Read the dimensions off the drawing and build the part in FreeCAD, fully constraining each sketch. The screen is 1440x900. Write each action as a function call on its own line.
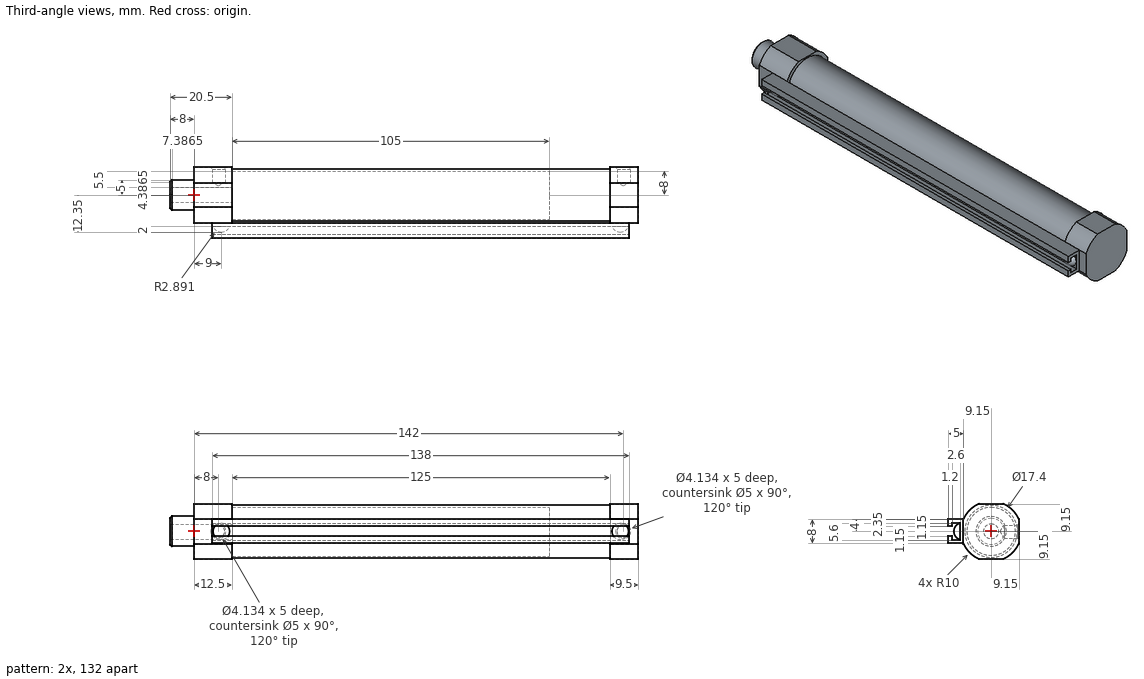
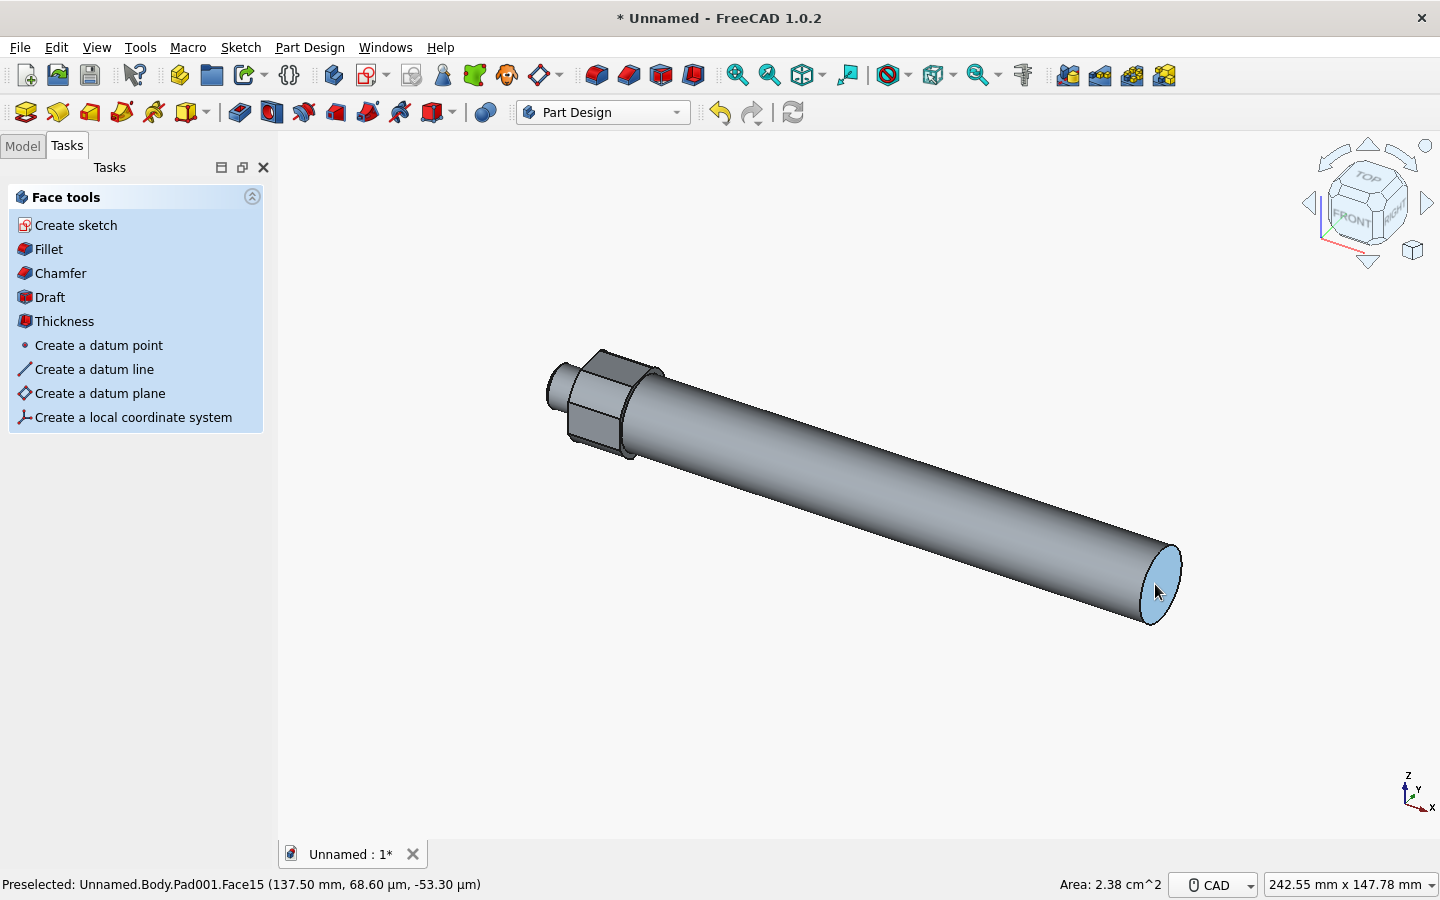
click(366, 76)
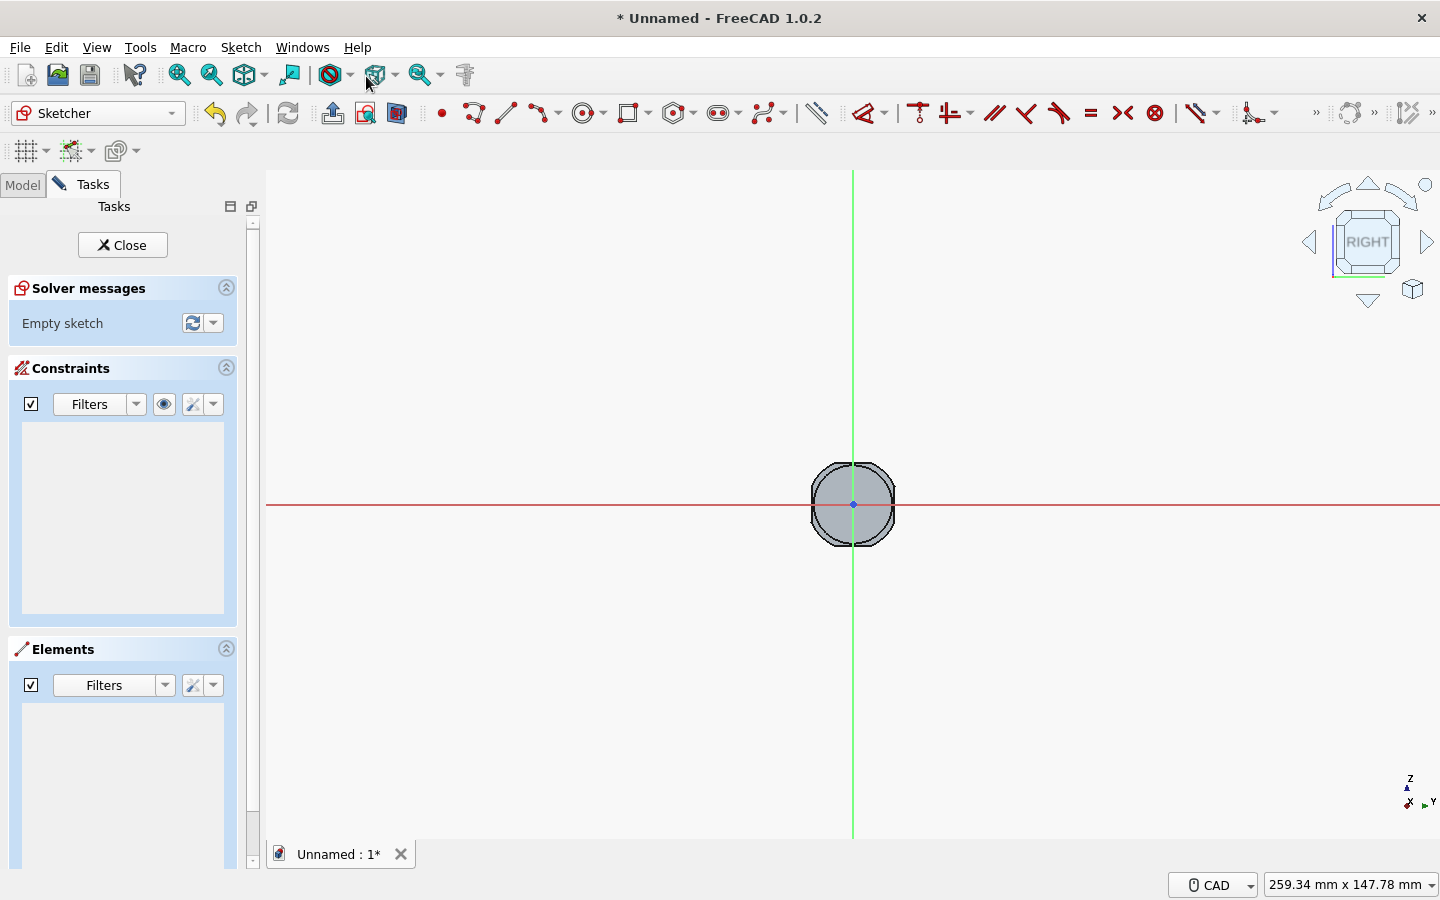
scroll(870, 504, up, 8)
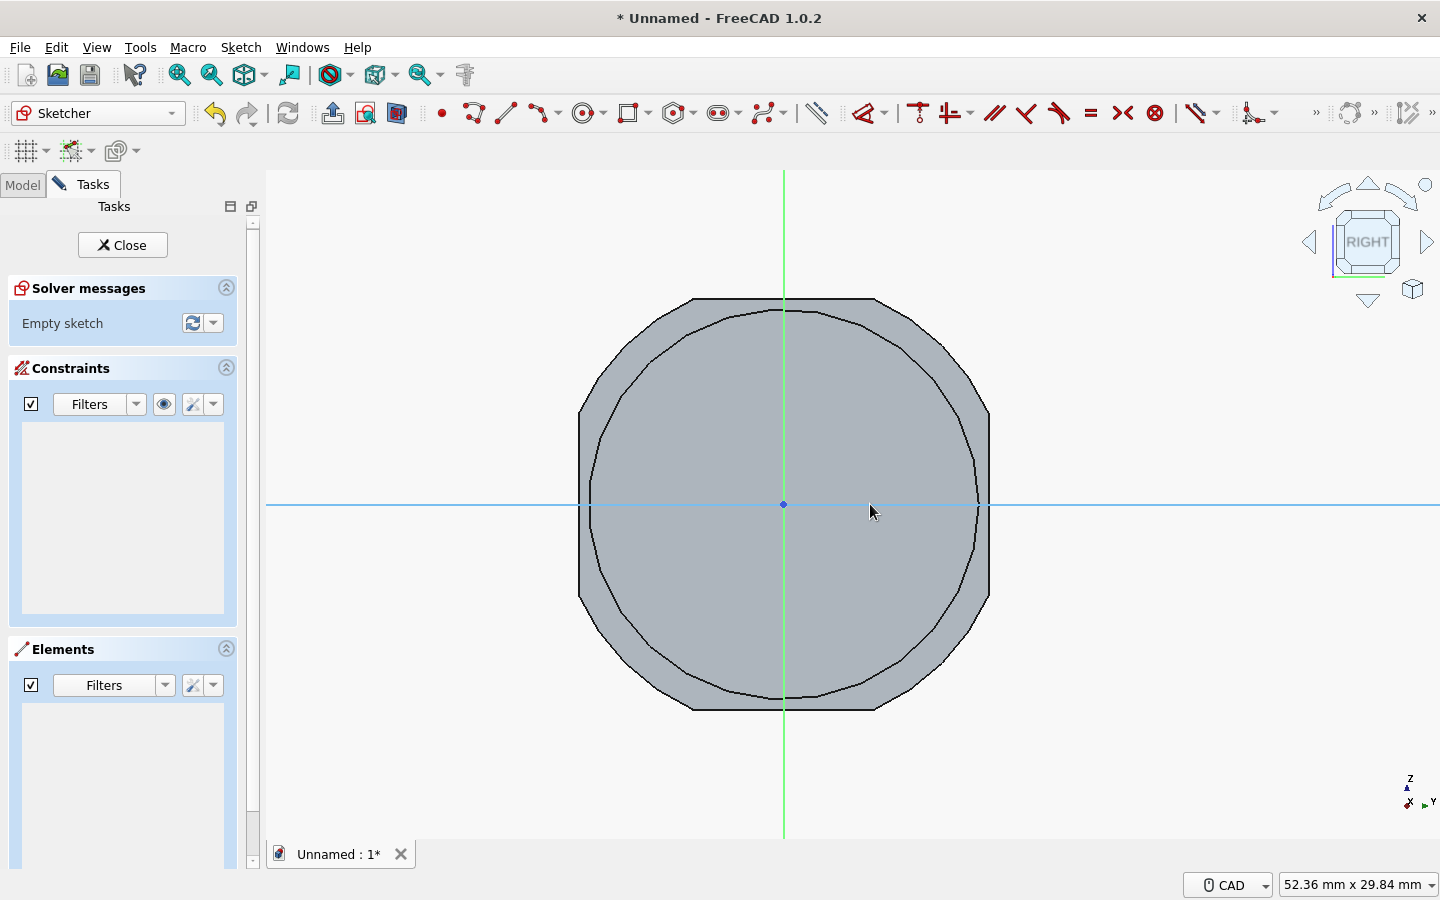
click(506, 114)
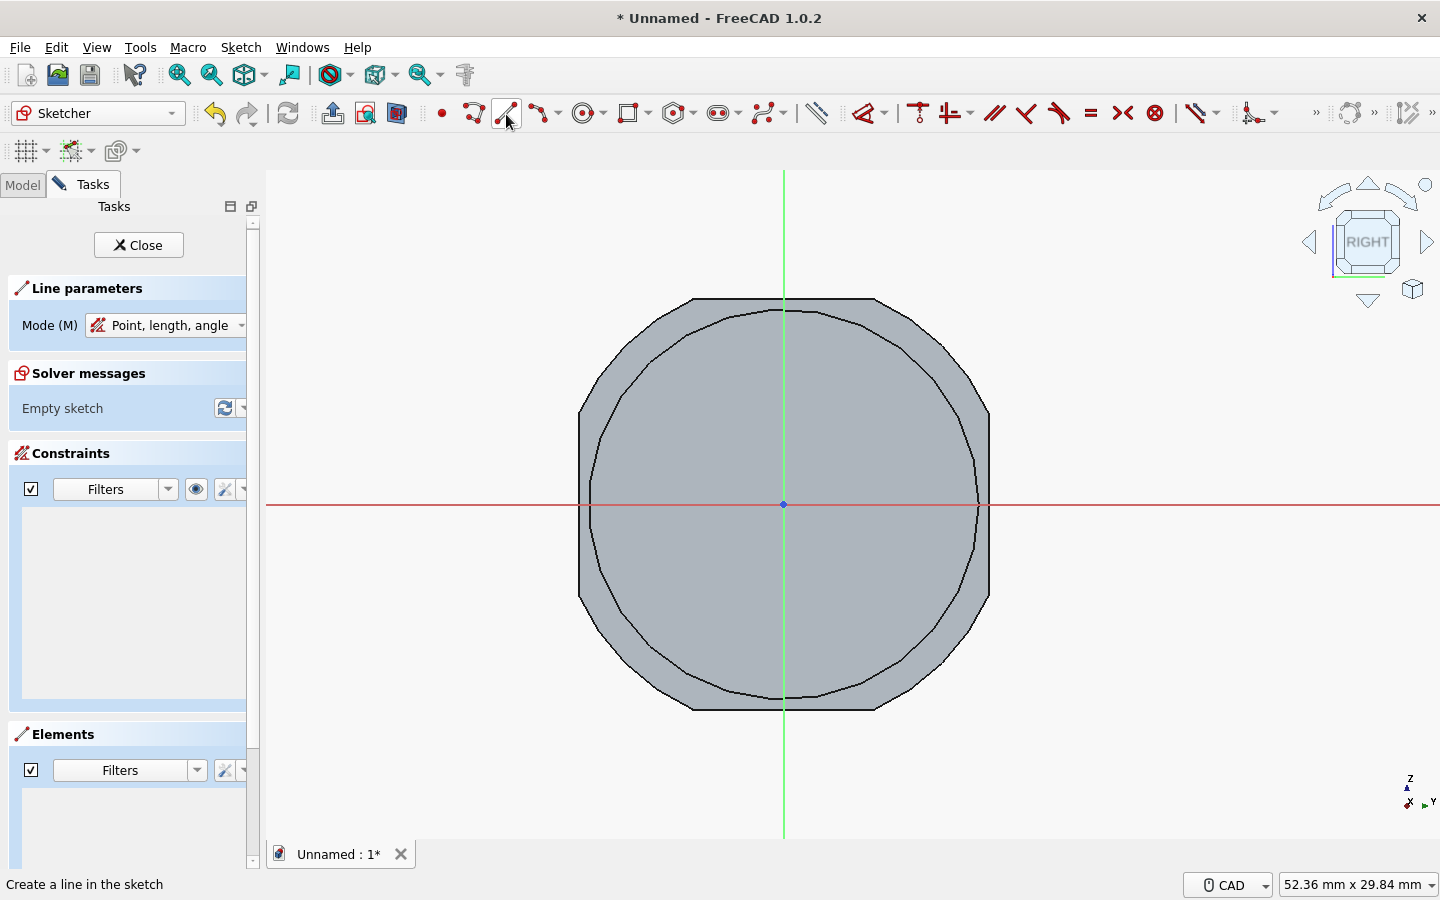
click(579, 414)
click(579, 595)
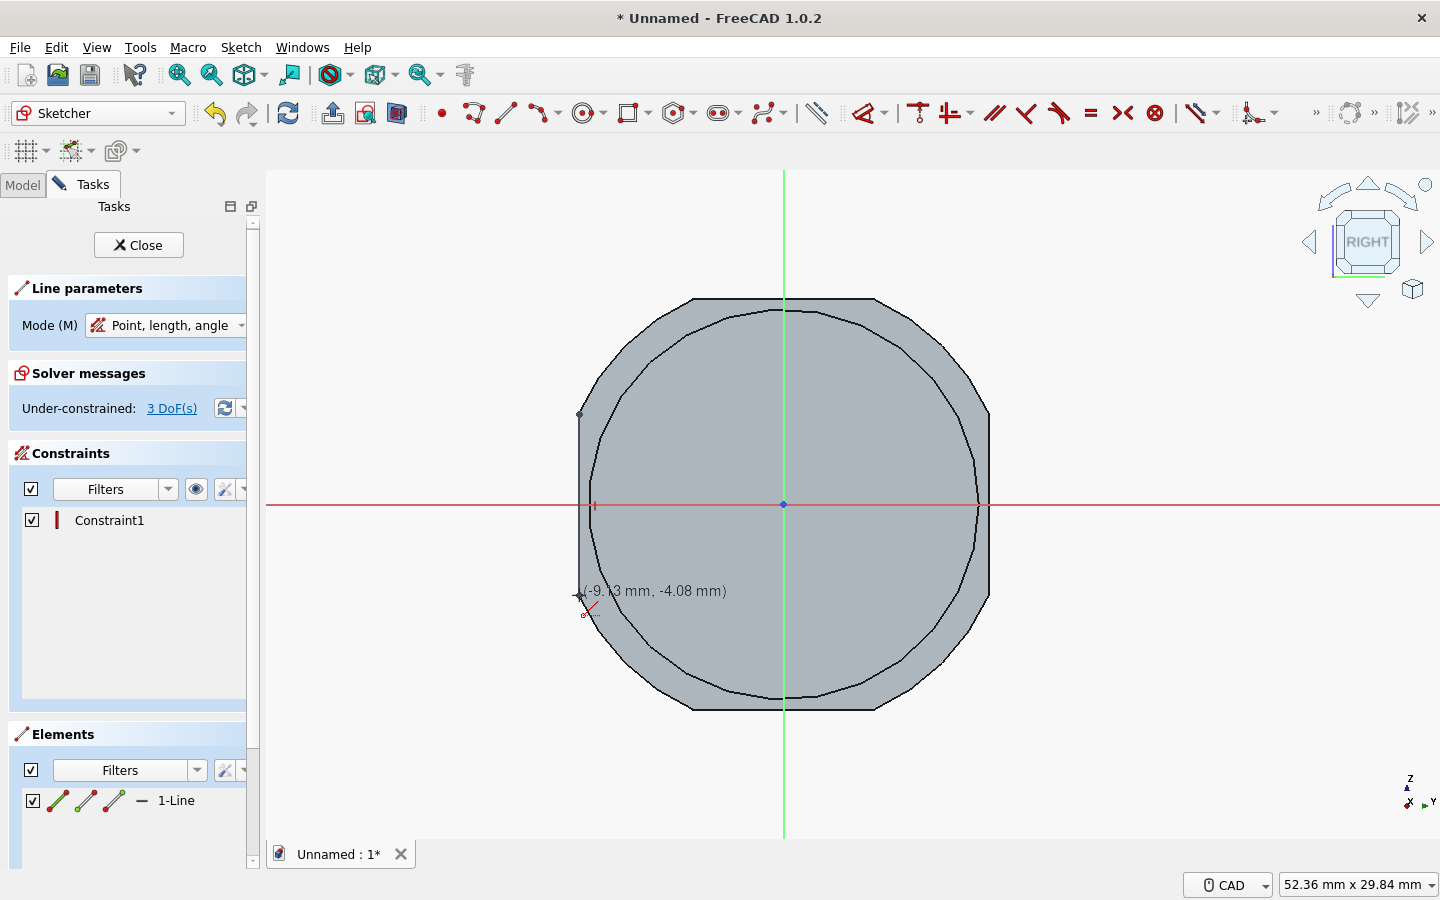
click(693, 710)
click(874, 710)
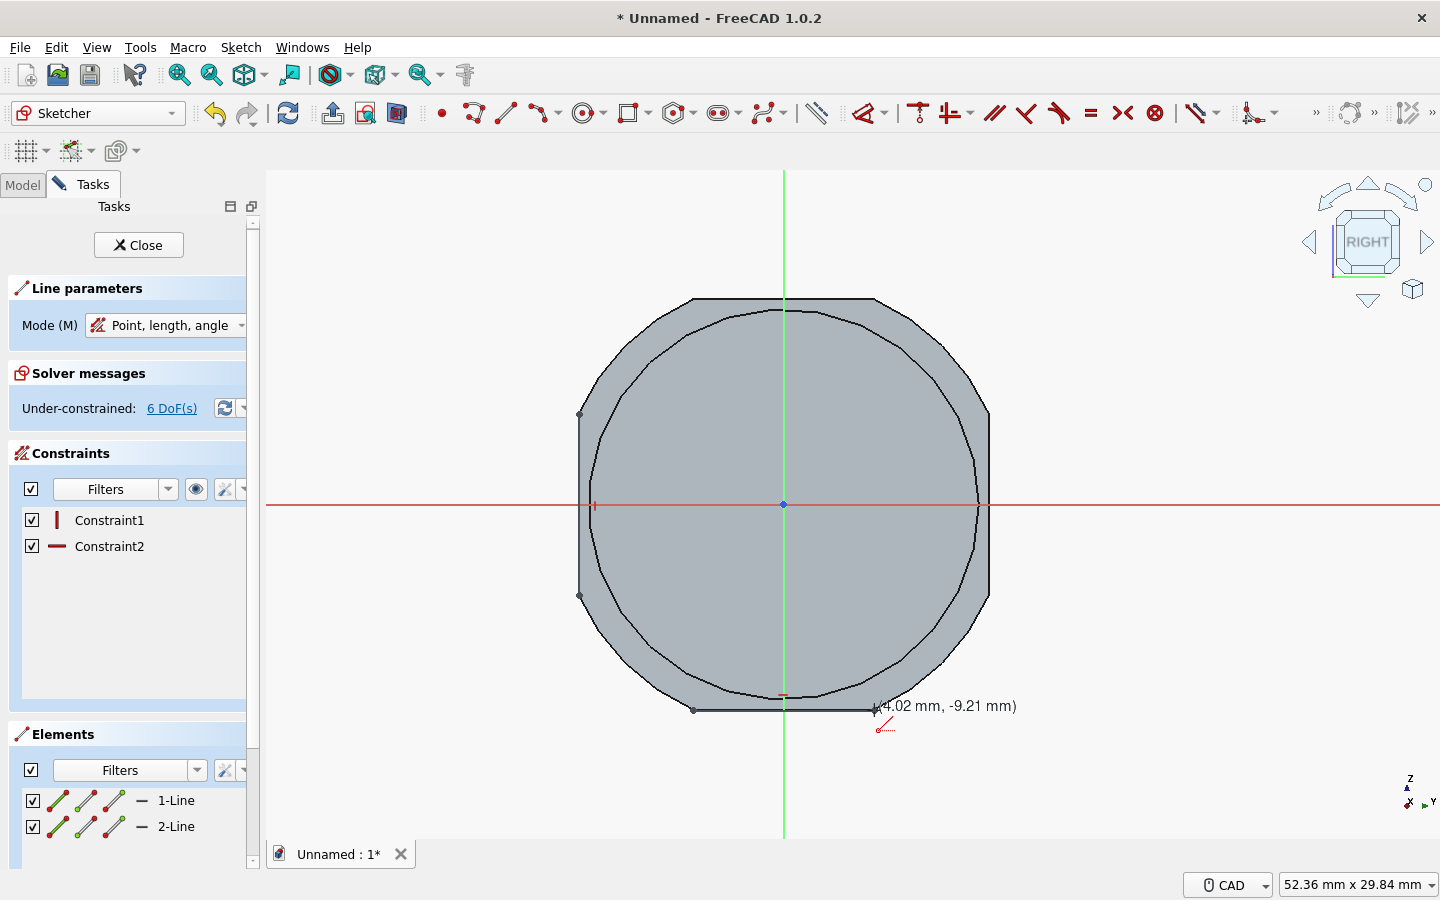
click(989, 595)
click(989, 414)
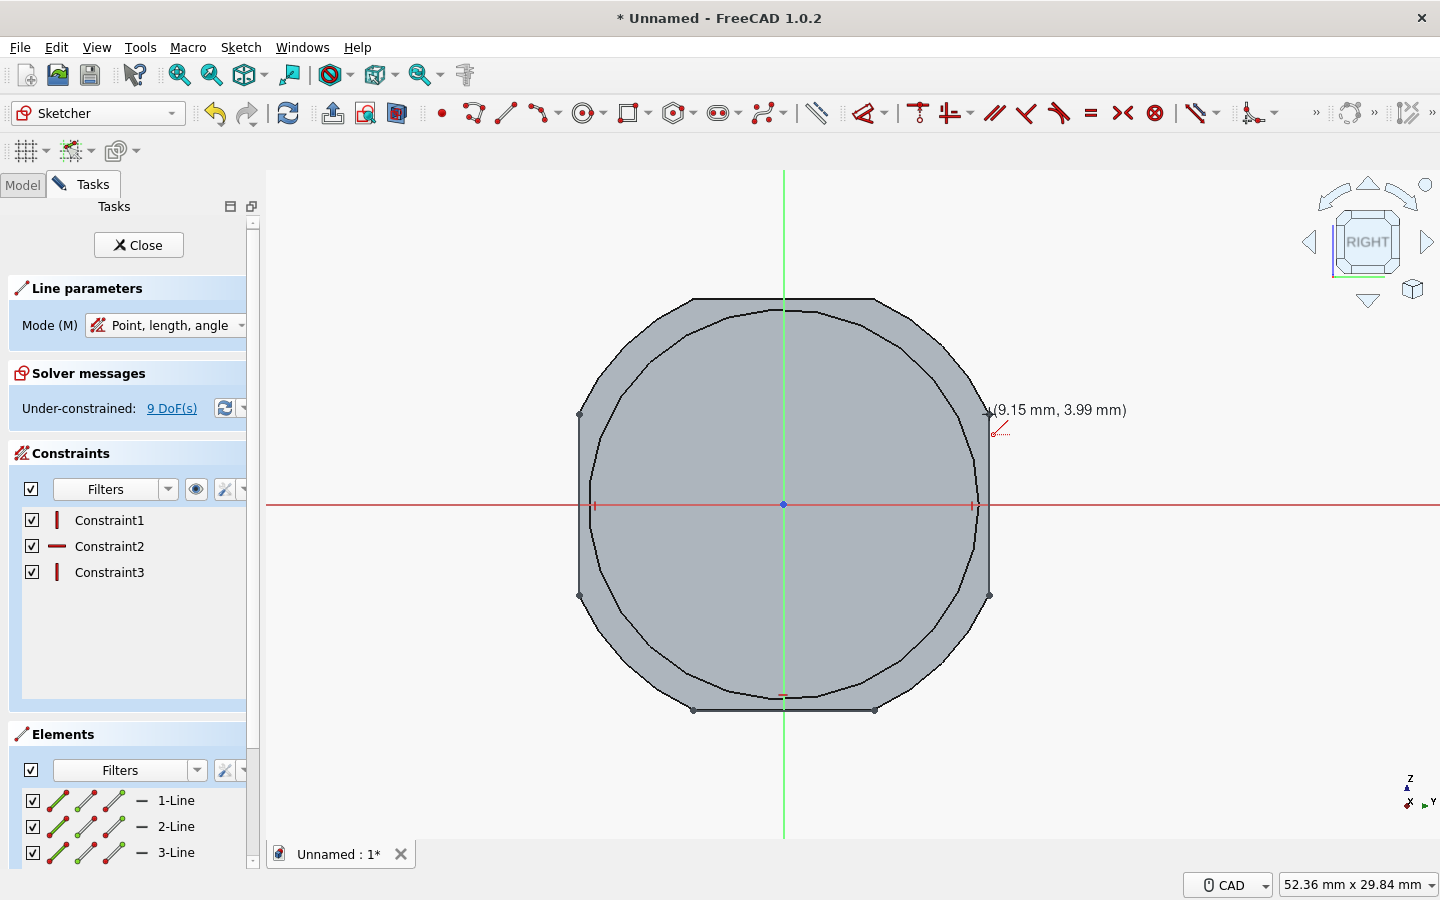
click(874, 299)
click(693, 299)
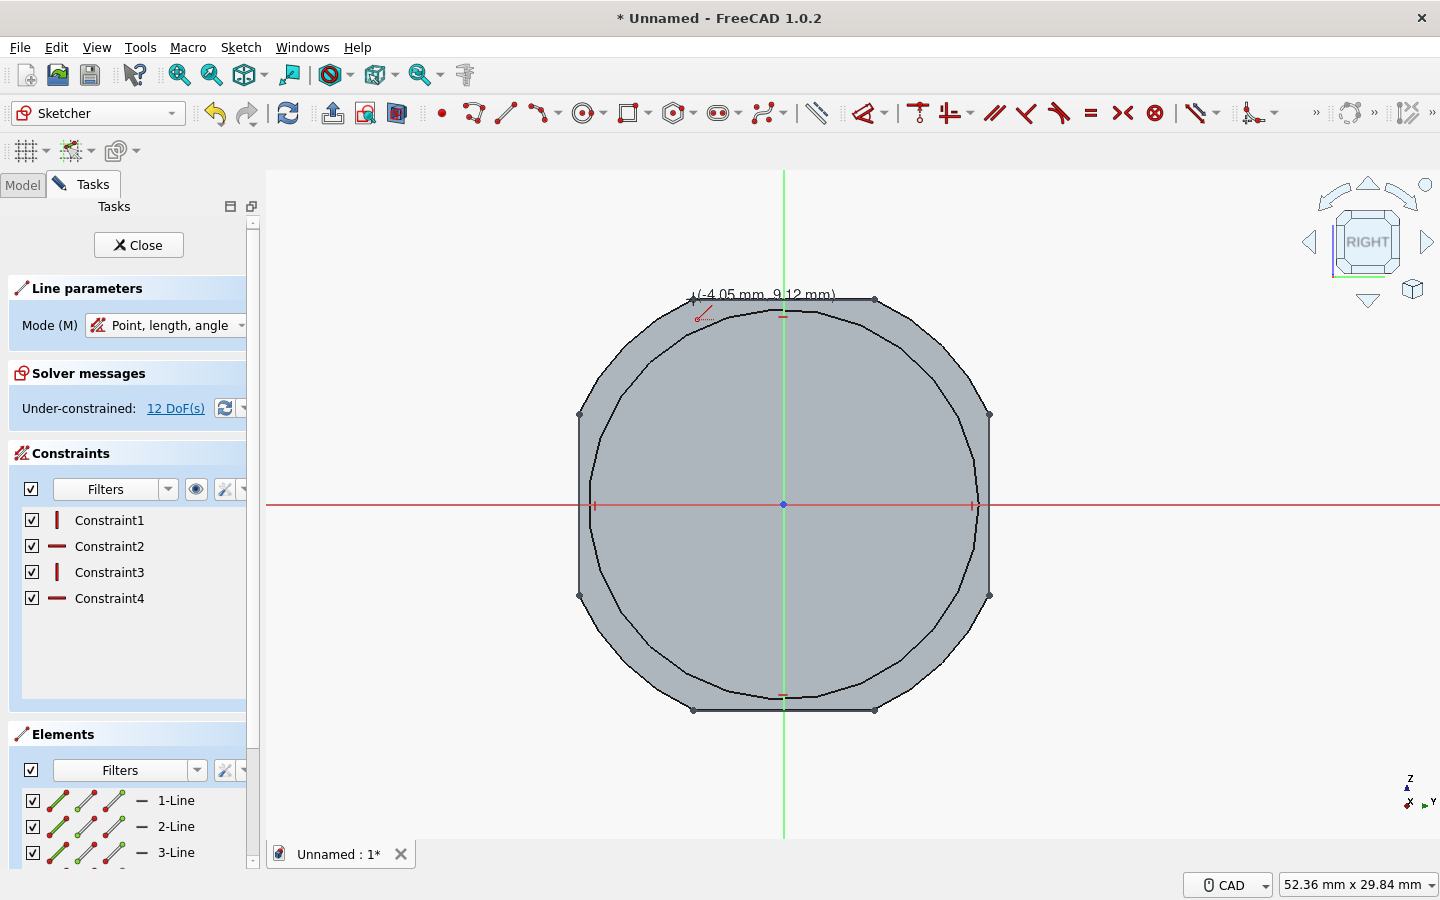
click(538, 114)